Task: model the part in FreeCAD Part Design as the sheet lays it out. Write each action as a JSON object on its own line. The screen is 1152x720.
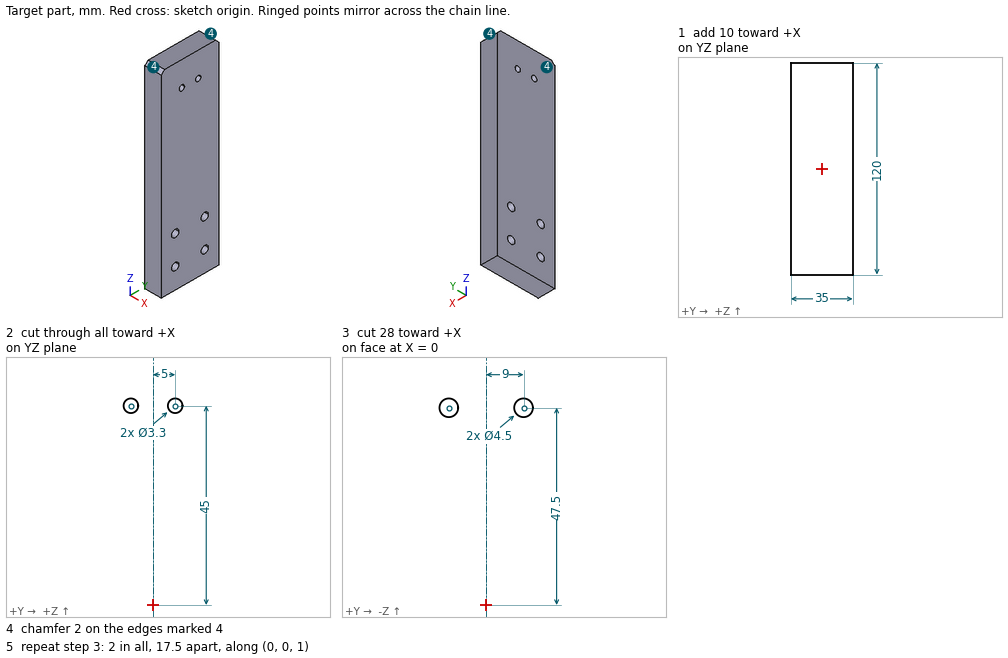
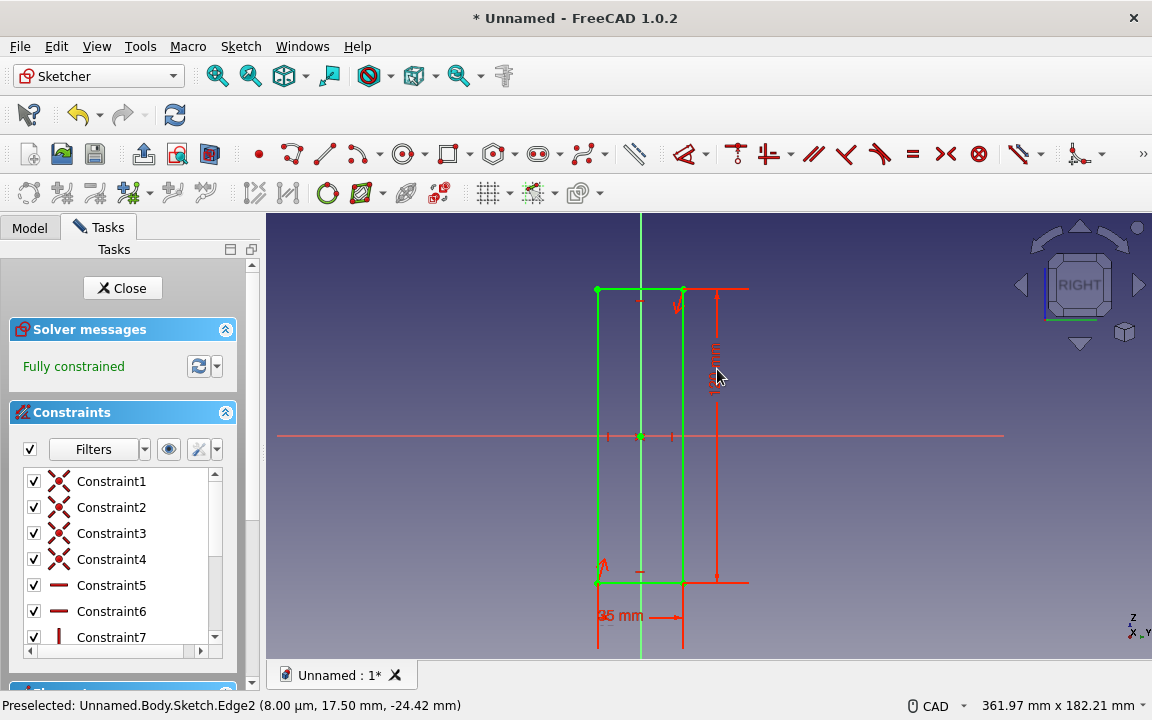
{"action": "left_click", "coordinate": [123, 288]}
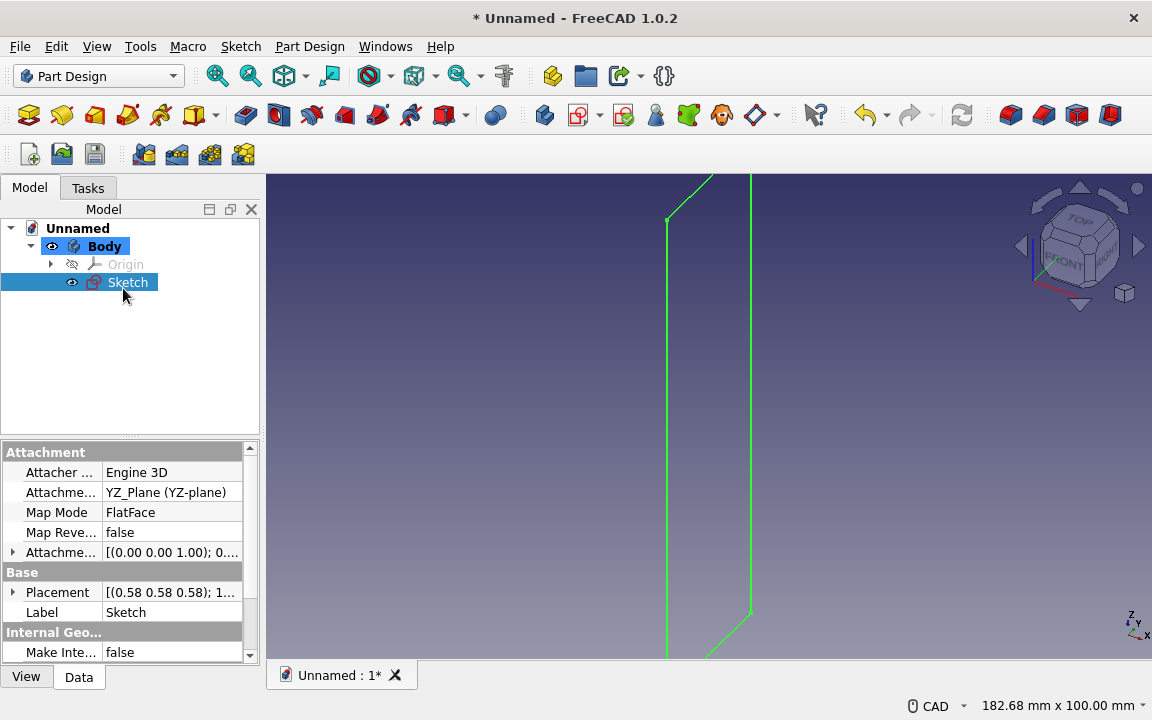
{"action": "left_click", "coordinate": [29, 116]}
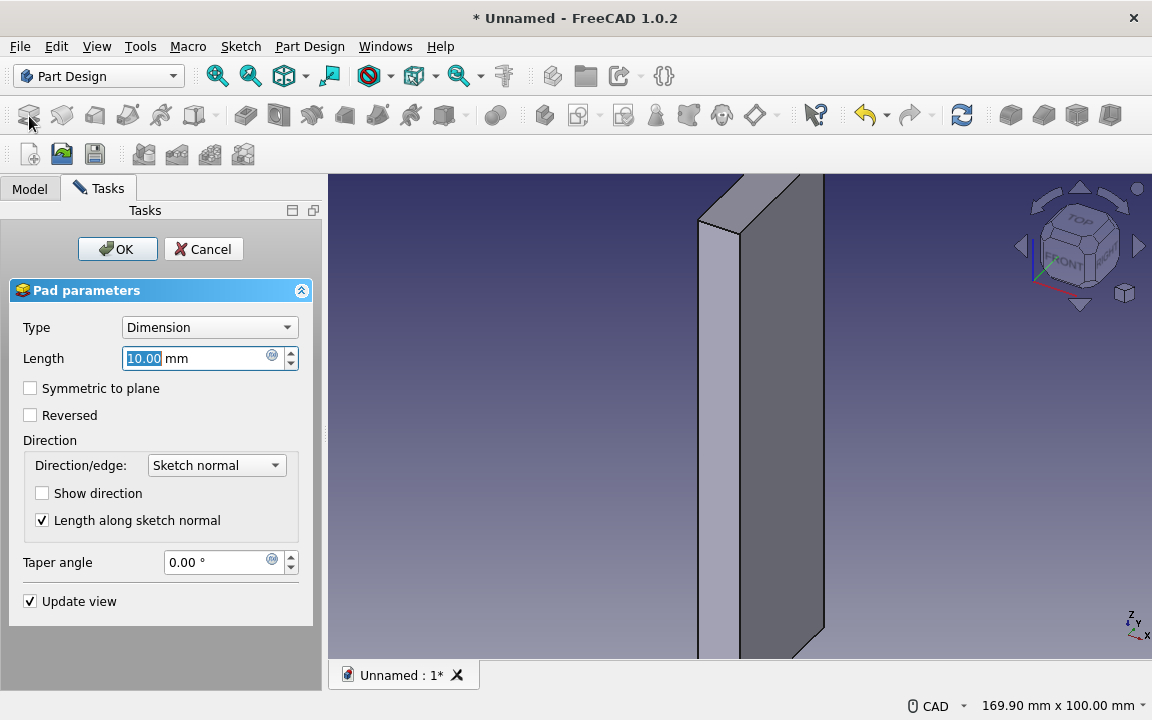
{"action": "type", "text": "10"}
{"action": "key", "text": "Tab"}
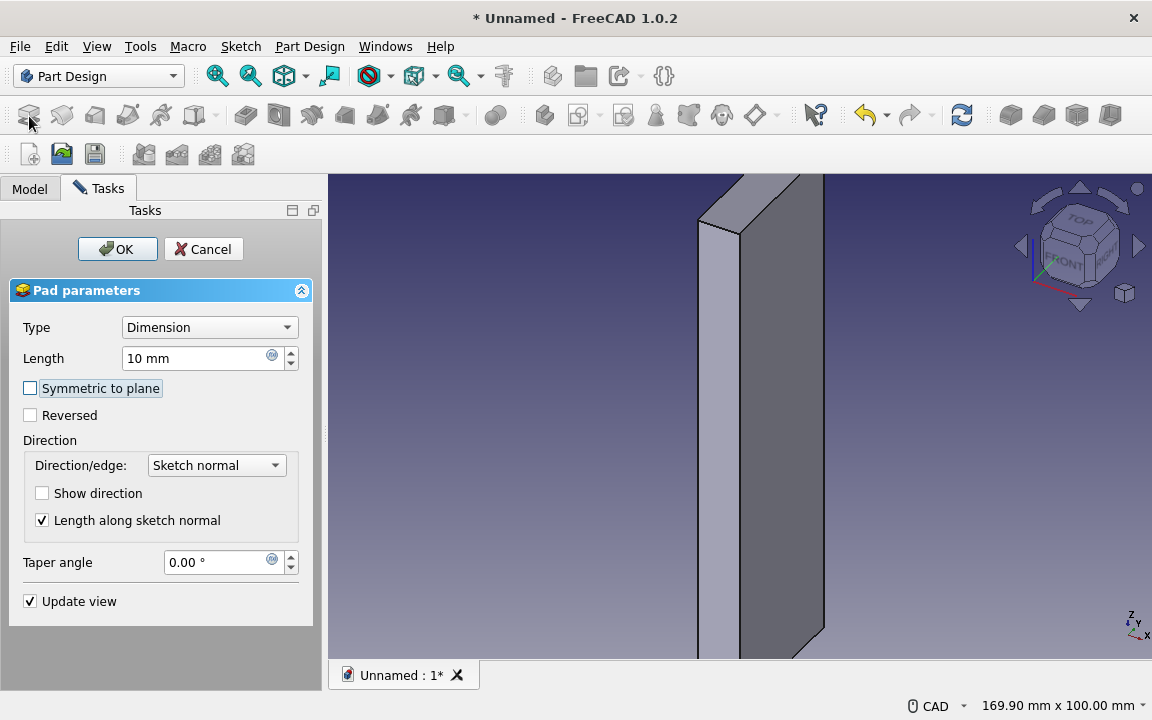
{"action": "left_click", "coordinate": [118, 249]}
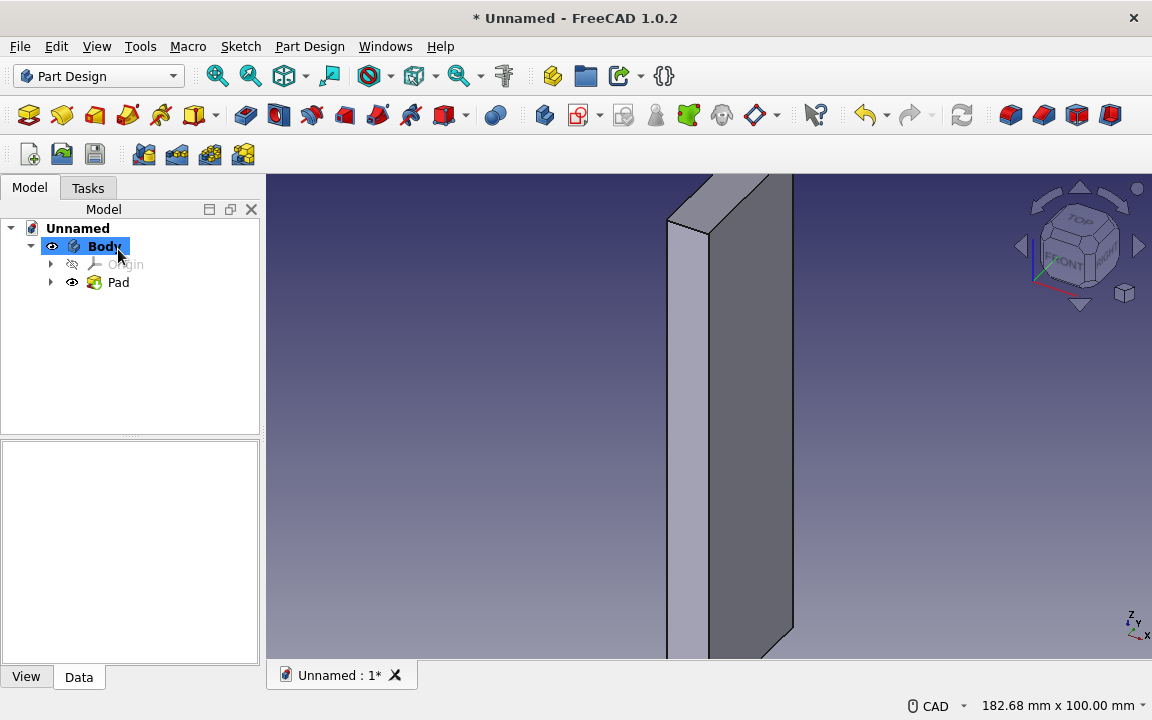
{"action": "left_click", "coordinate": [218, 76]}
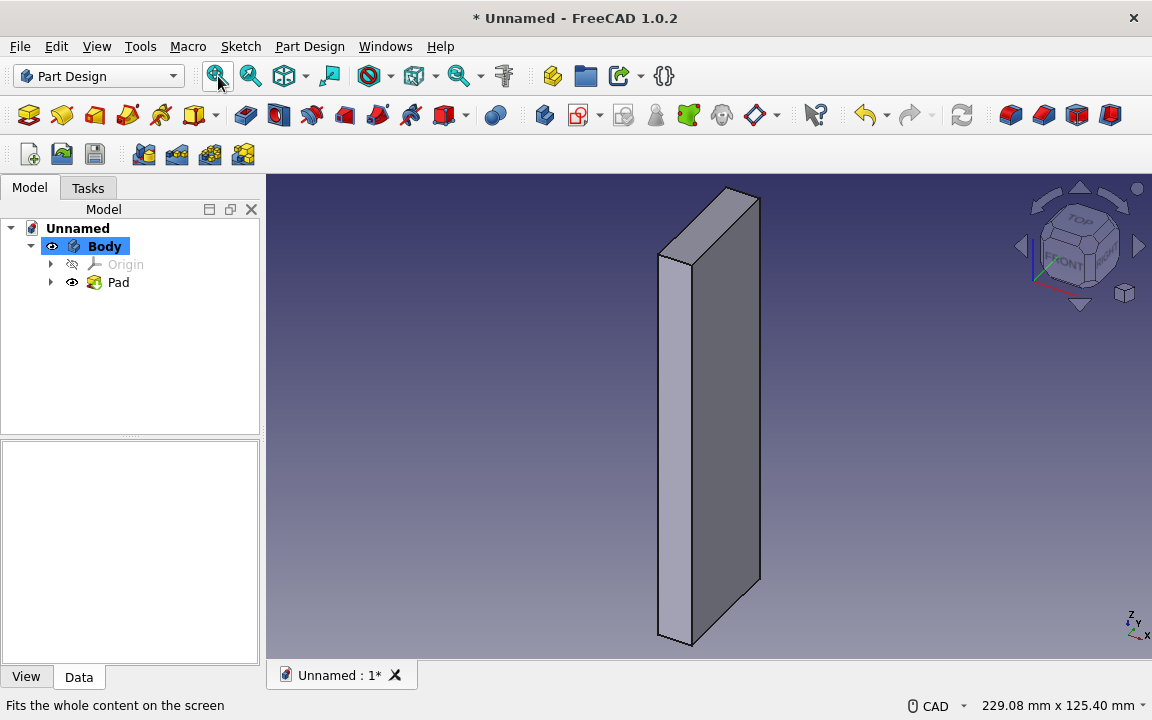
{"action": "left_click", "coordinate": [578, 116]}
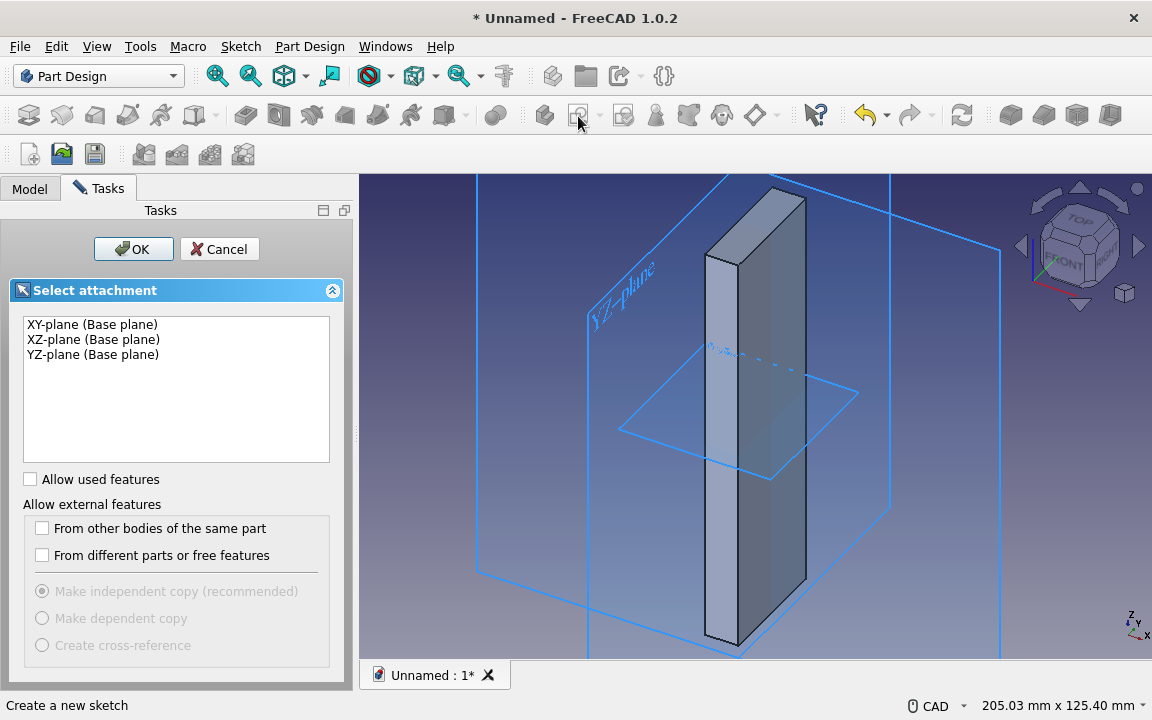
{"action": "left_click", "coordinate": [84, 354]}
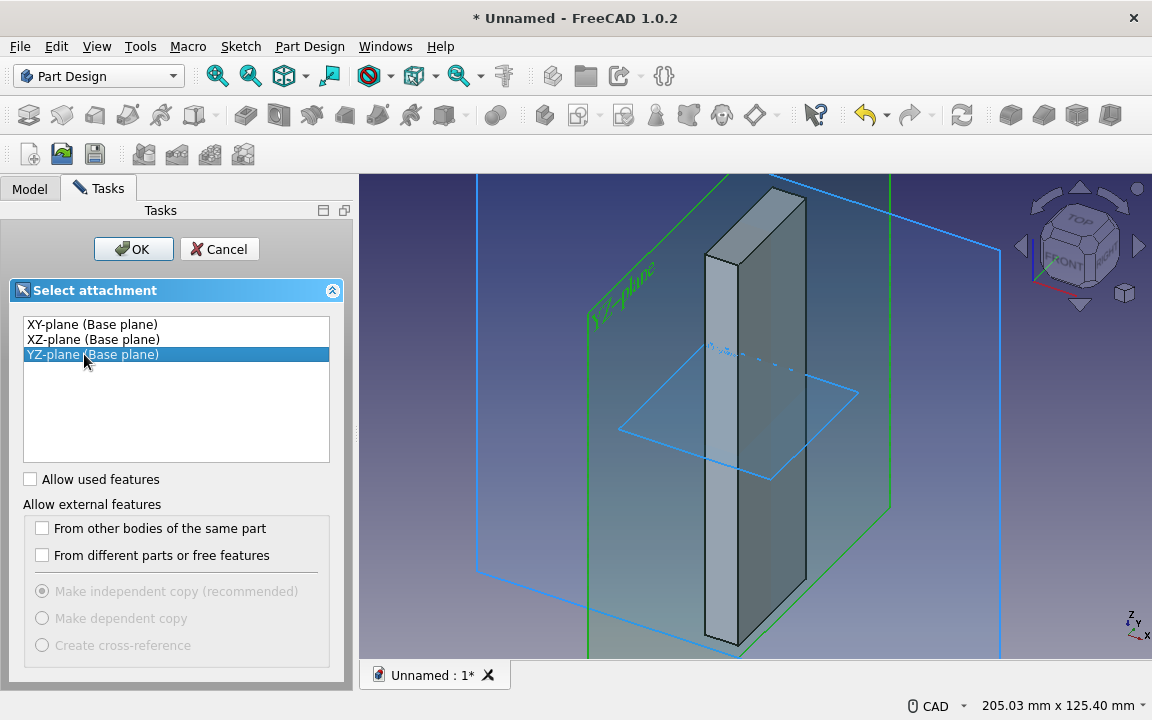
{"action": "left_click", "coordinate": [134, 249]}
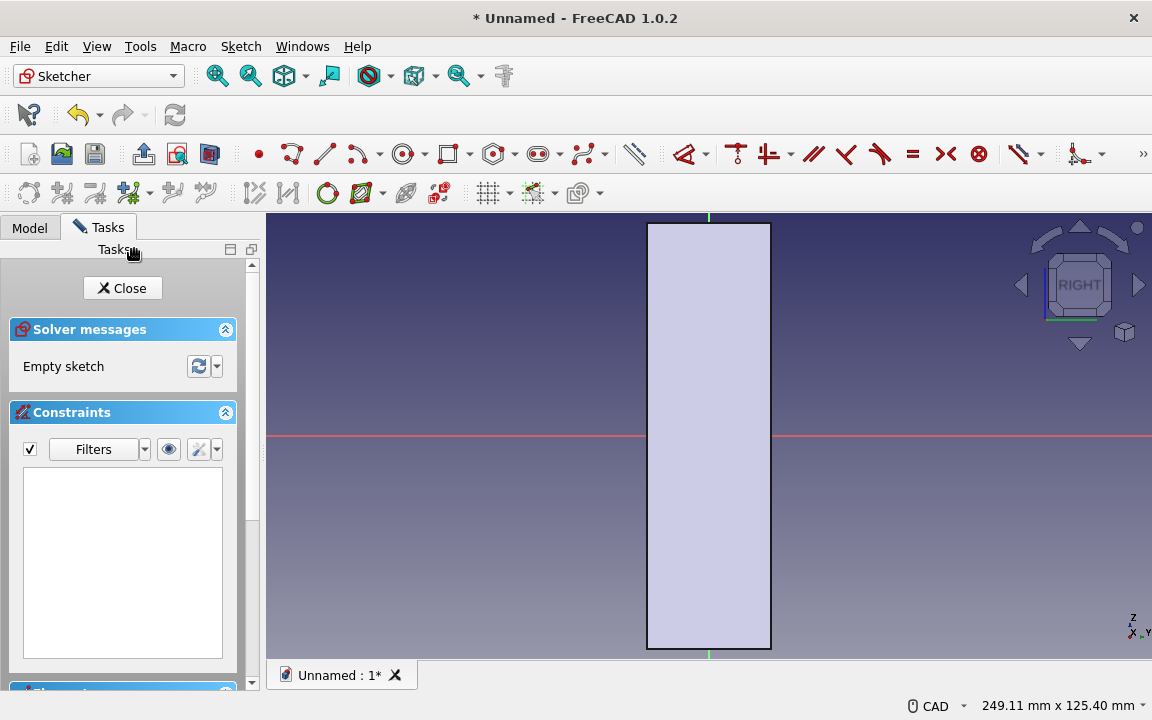
{"action": "left_click", "coordinate": [210, 154]}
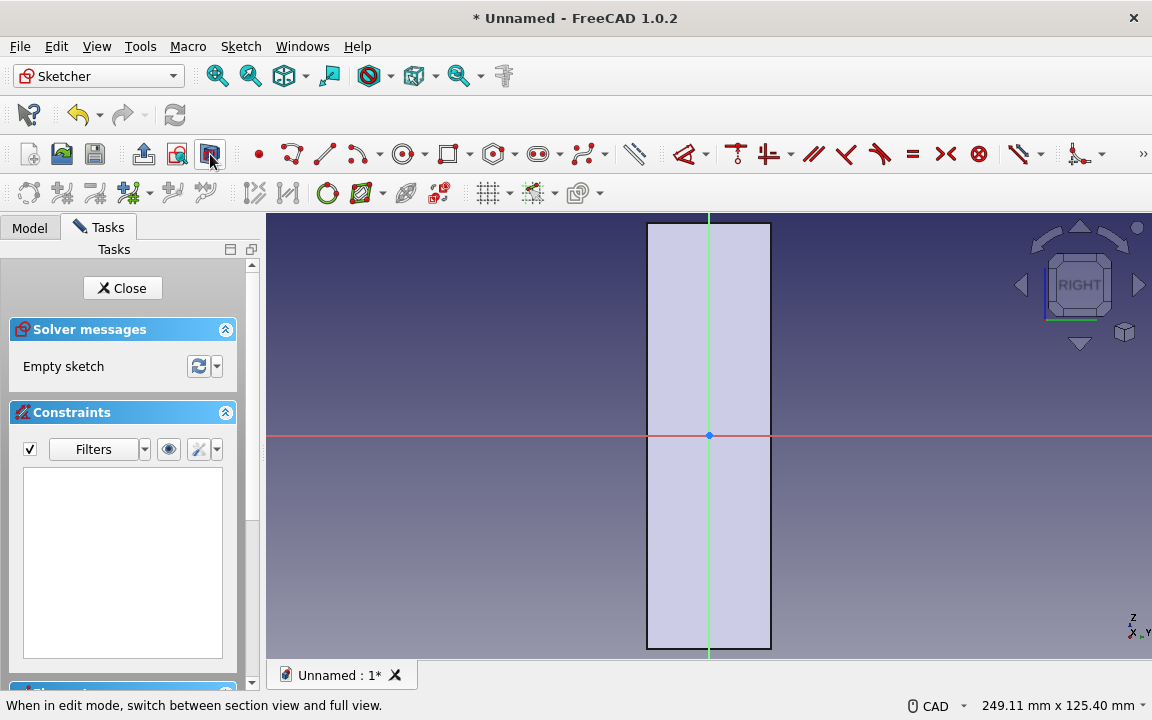
{"action": "scroll", "coordinate": [716, 260], "scroll_direction": "up", "scroll_amount": 12}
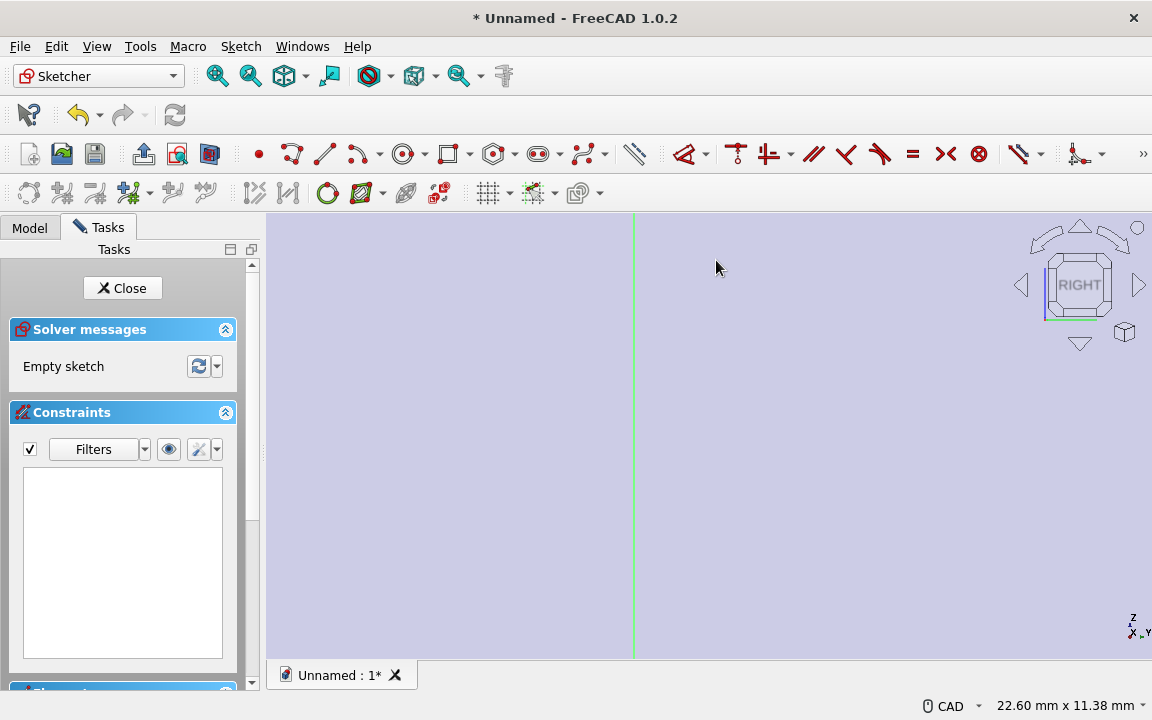
{"action": "left_click", "coordinate": [402, 154]}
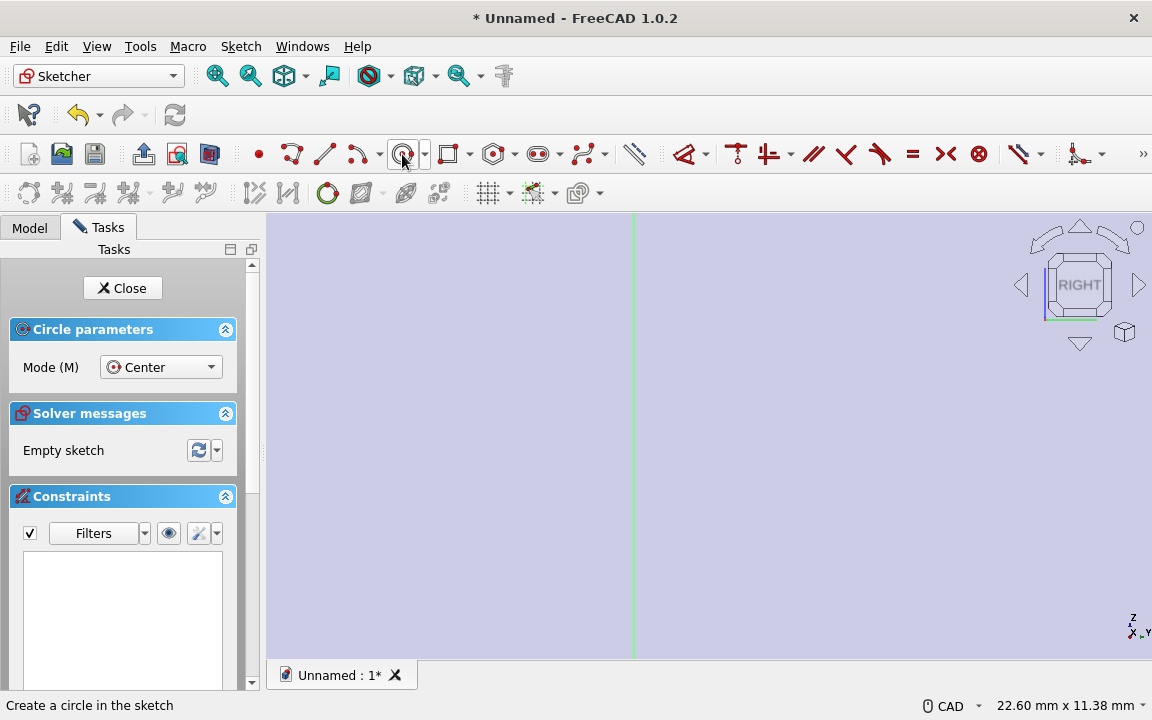
{"action": "left_click", "coordinate": [830, 435]}
{"action": "left_click", "coordinate": [876, 389]}